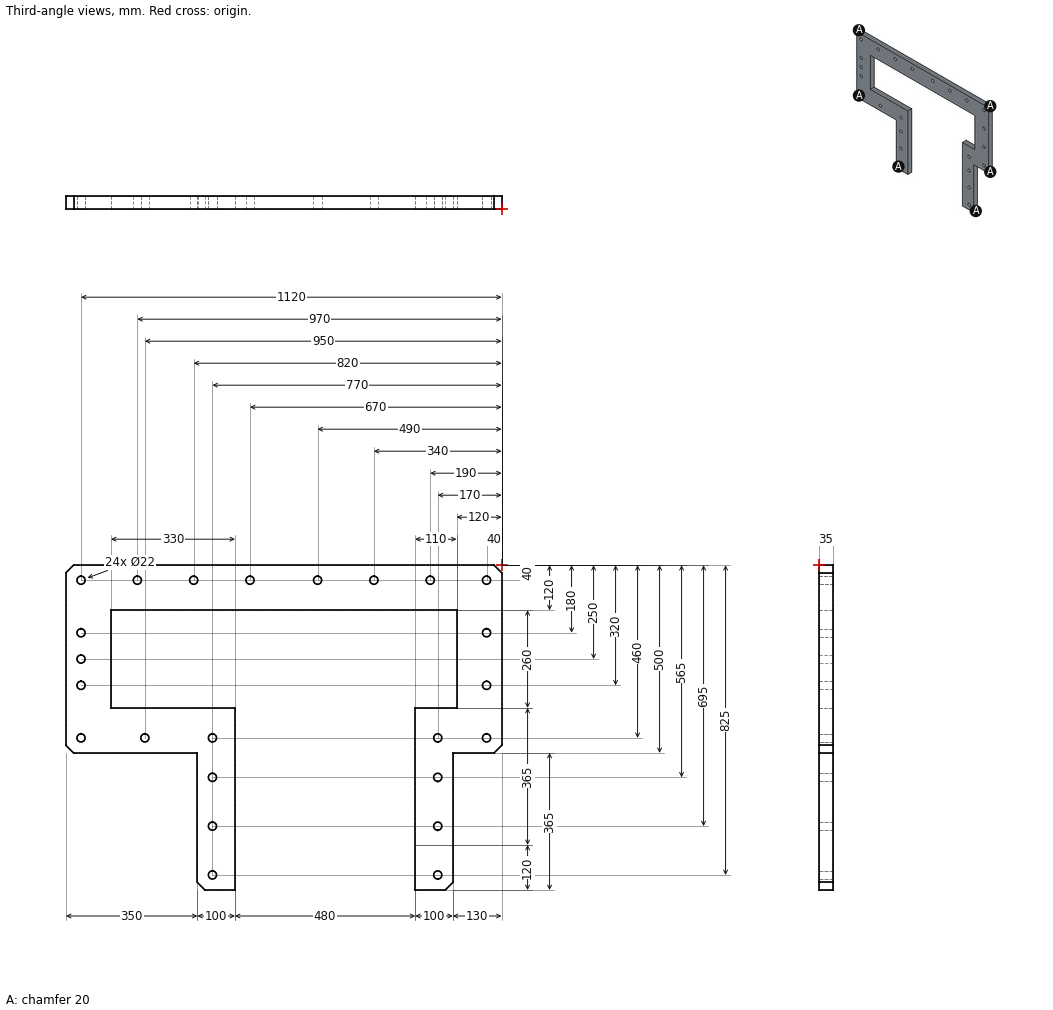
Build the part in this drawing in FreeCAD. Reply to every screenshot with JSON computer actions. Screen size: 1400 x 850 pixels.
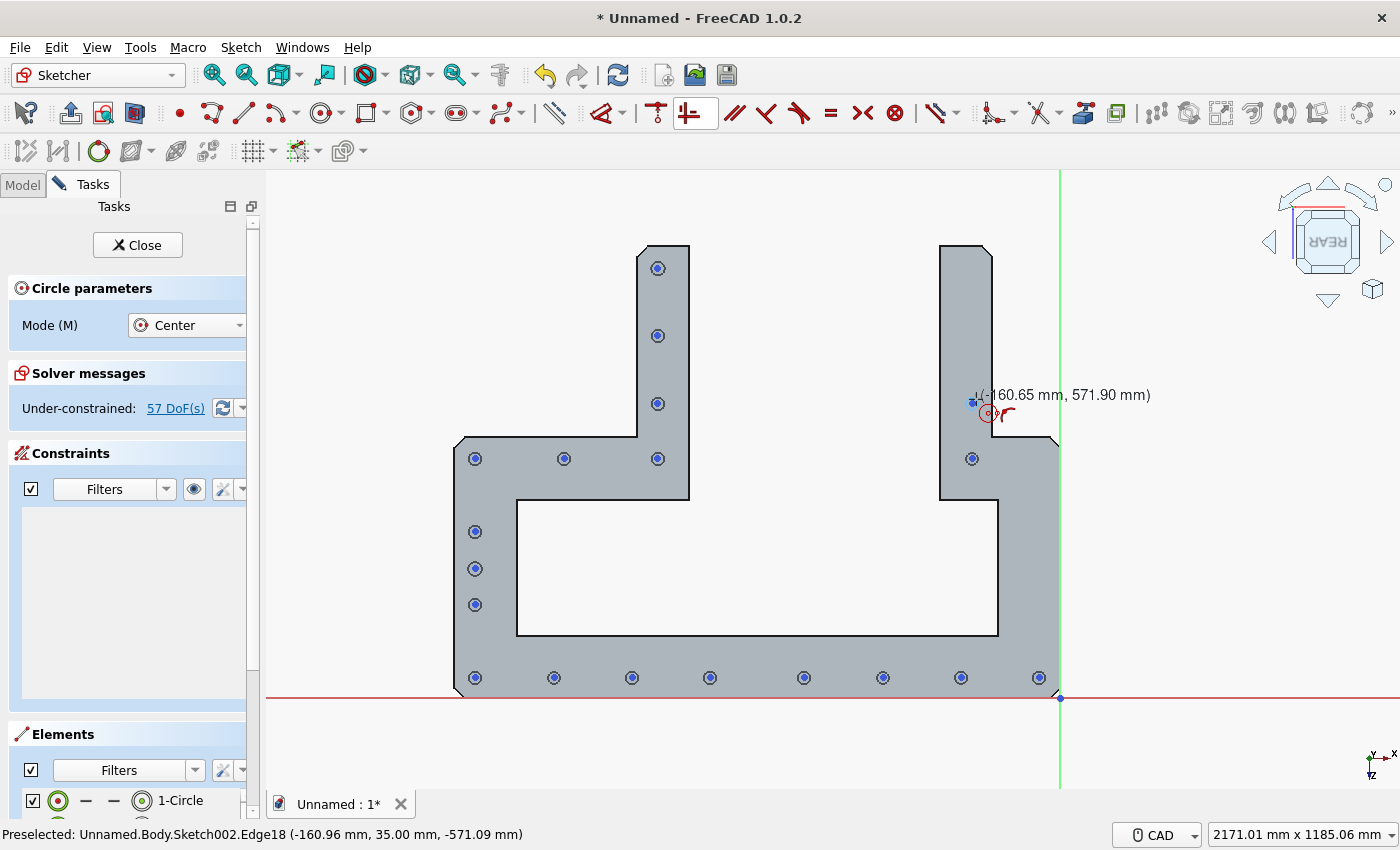
{"action": "scroll", "coordinate": [972, 335], "scroll_direction": "up", "scroll_amount": 7}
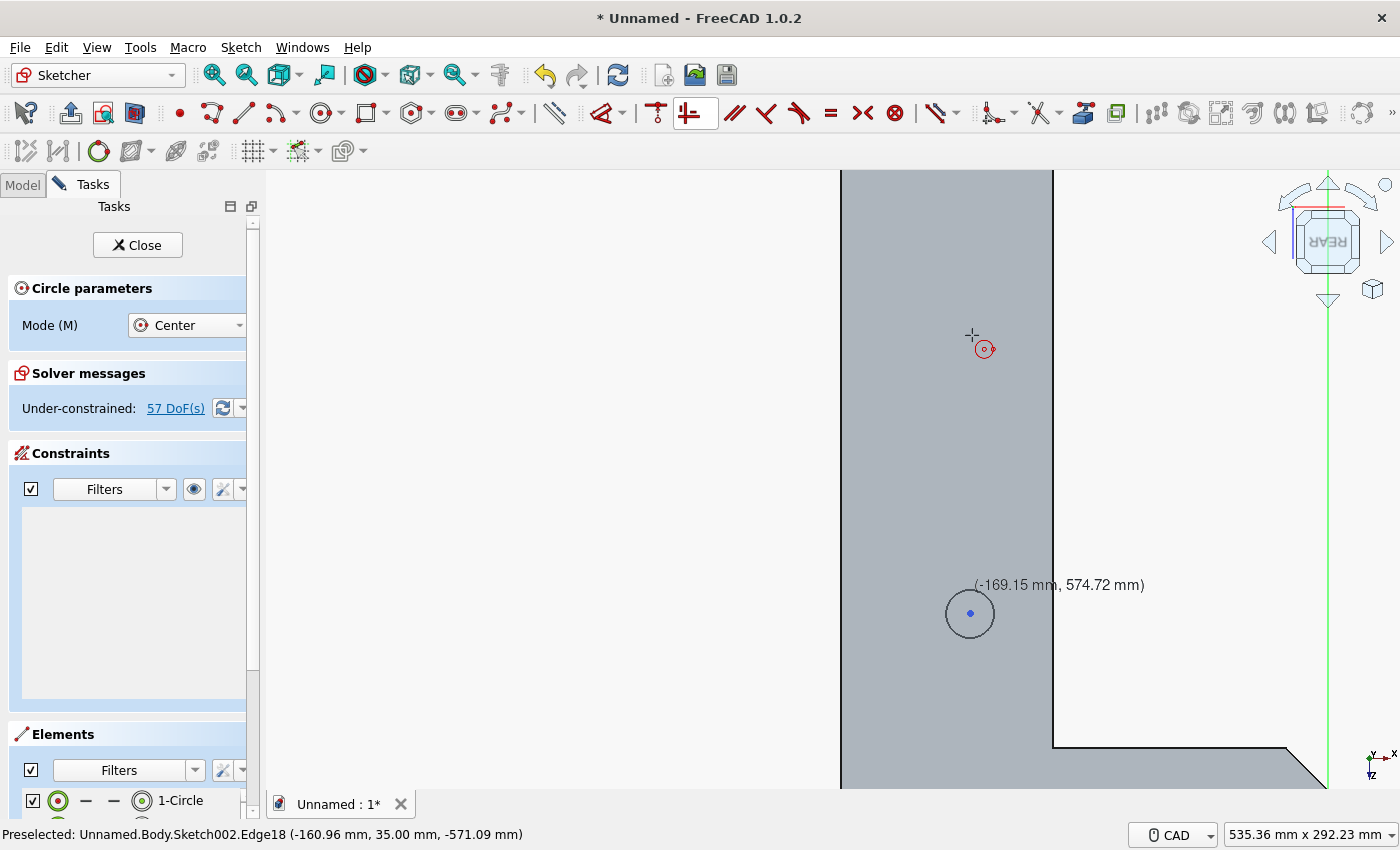
{"action": "scroll", "coordinate": [972, 335], "scroll_direction": "down", "scroll_amount": 7}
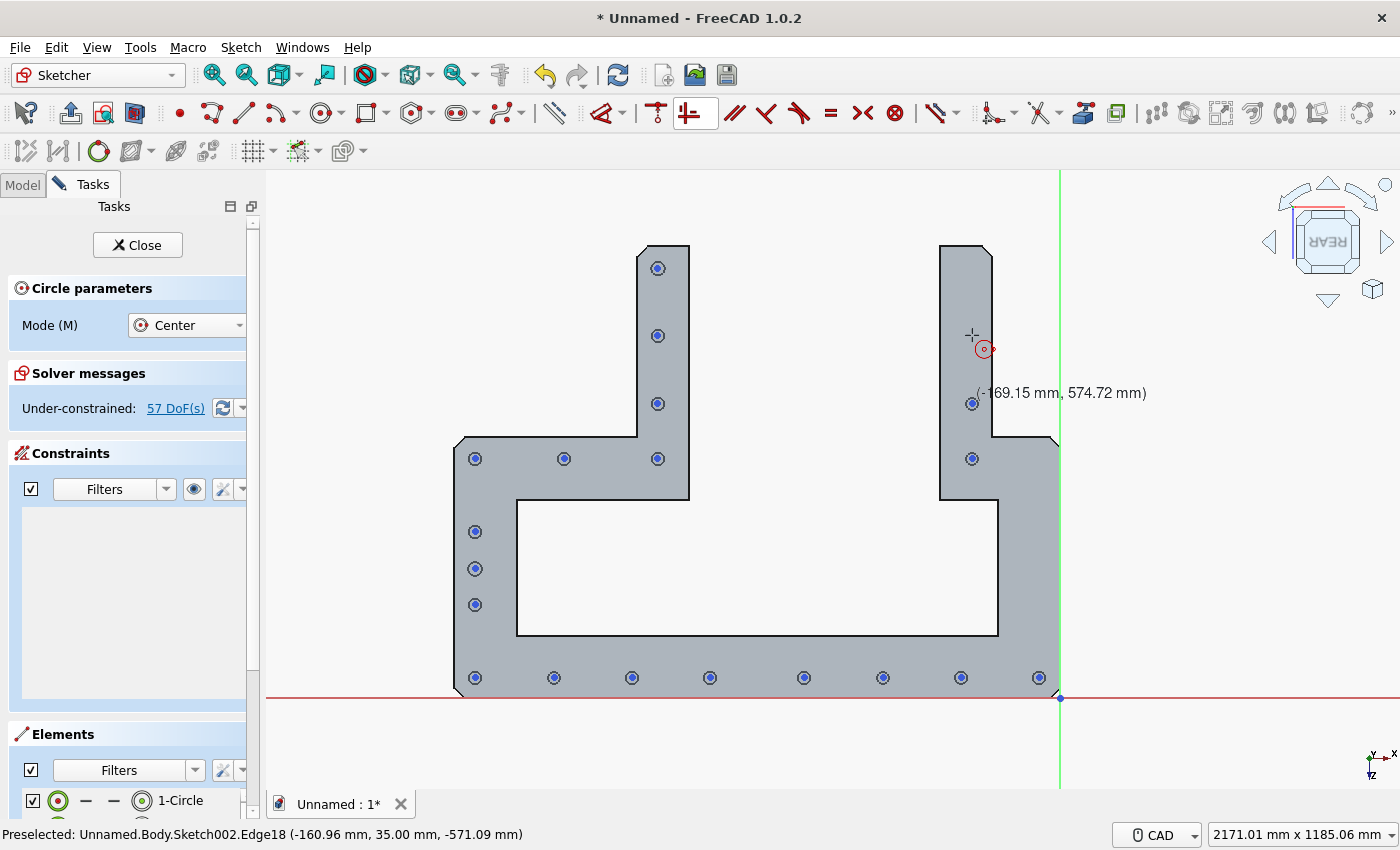
{"action": "left_click", "coordinate": [972, 335]}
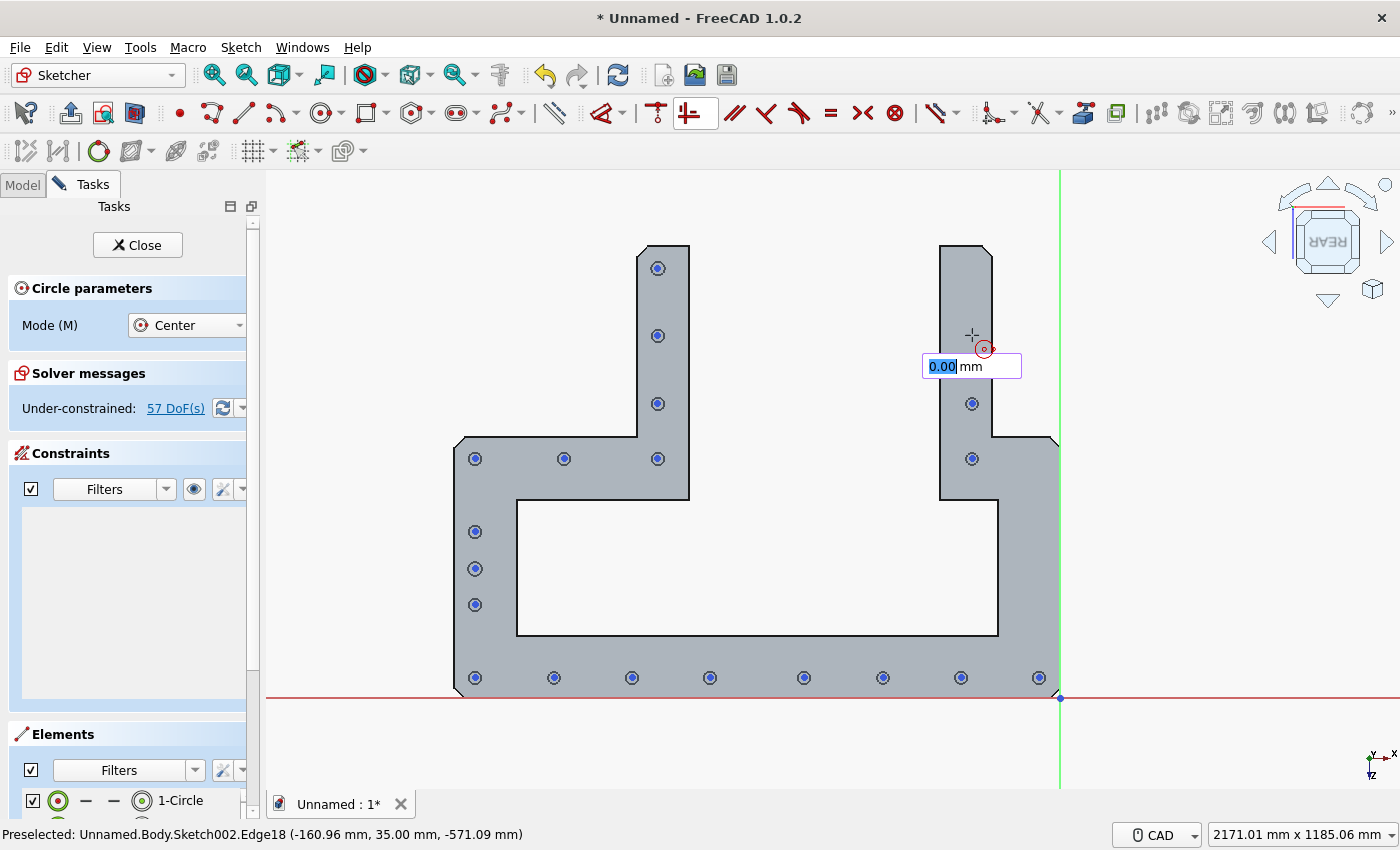
{"action": "scroll", "coordinate": [976, 331], "scroll_direction": "up", "scroll_amount": 6}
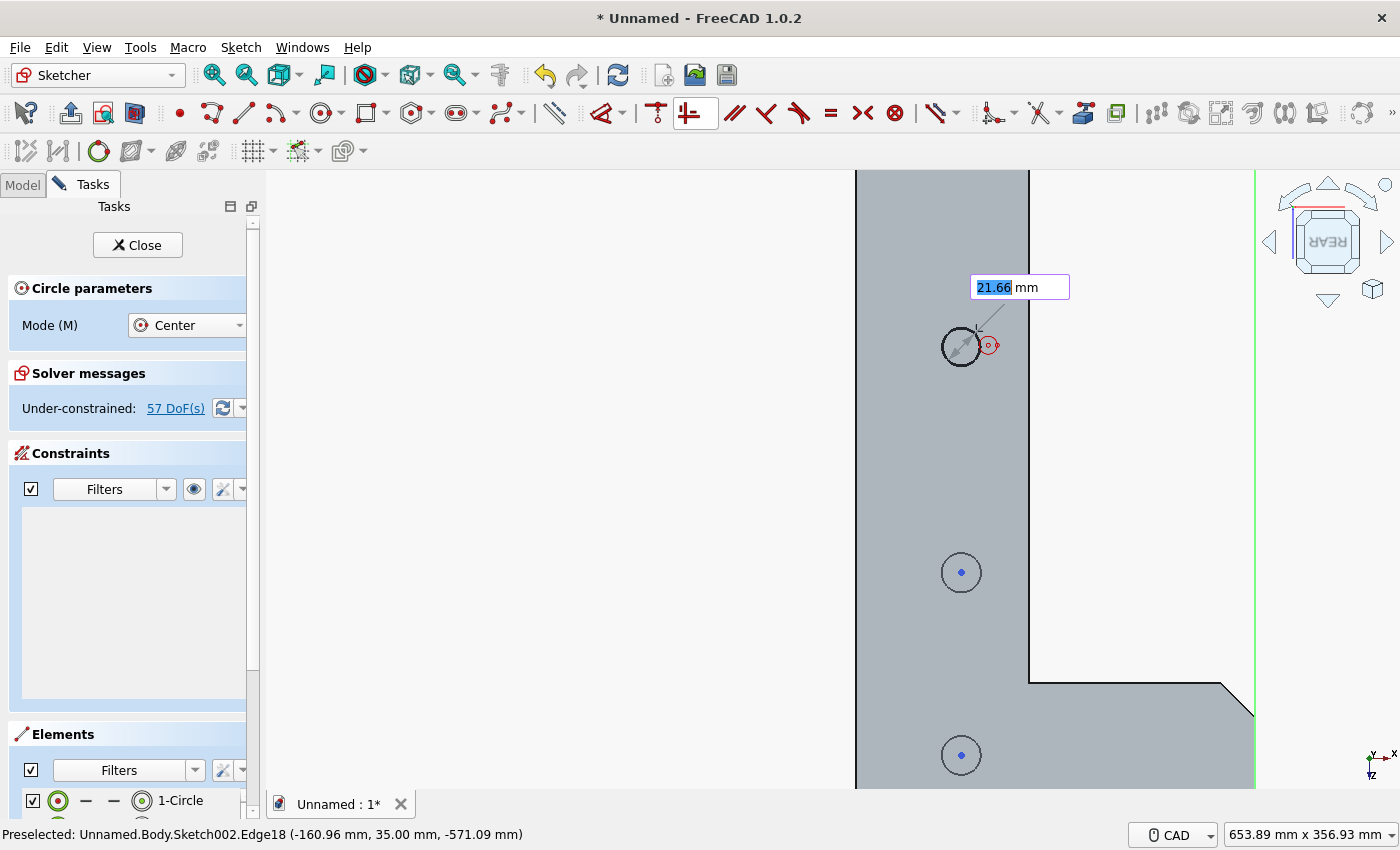
{"action": "left_click", "coordinate": [973, 331]}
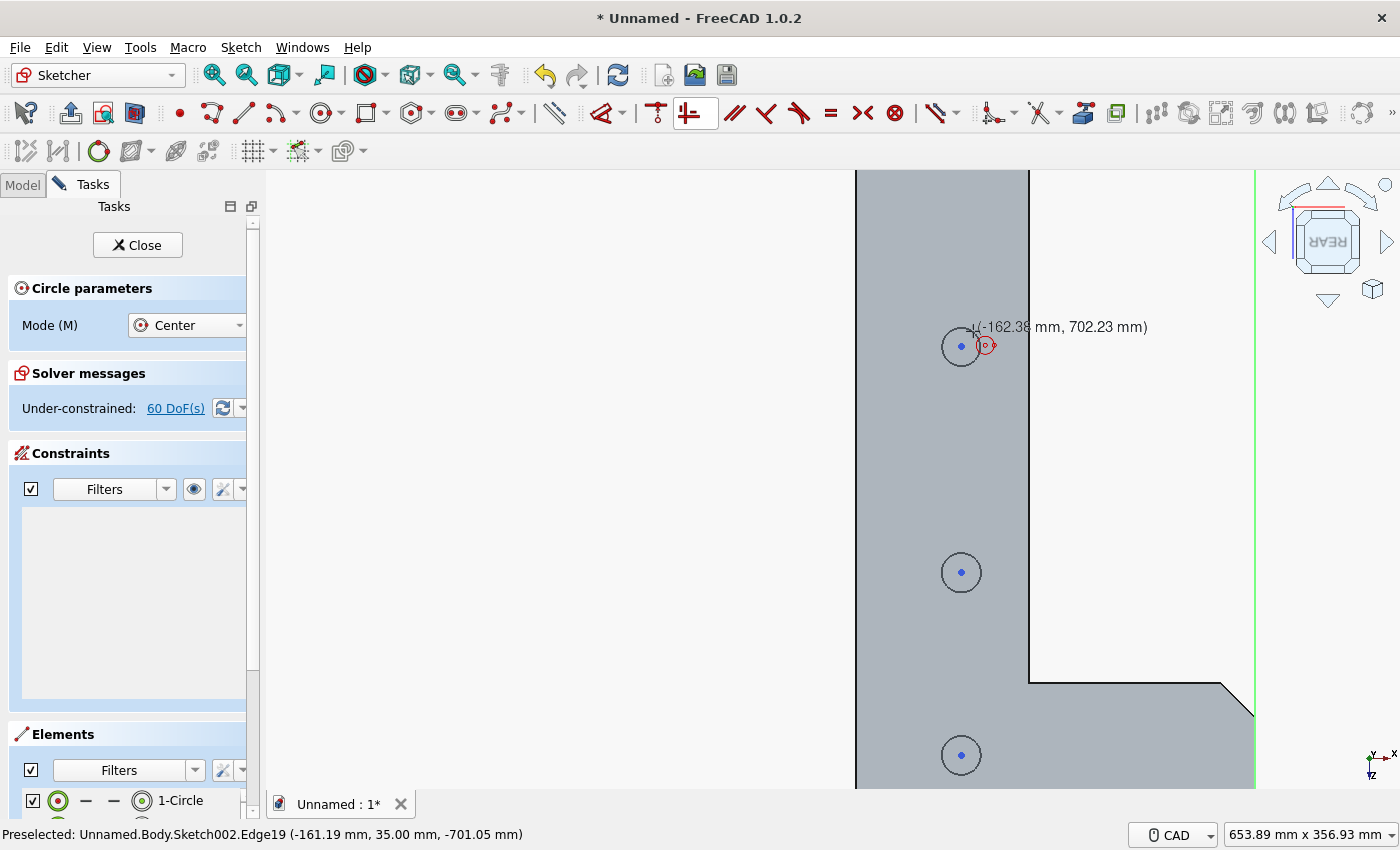
{"action": "scroll", "coordinate": [976, 331], "scroll_direction": "down", "scroll_amount": 6}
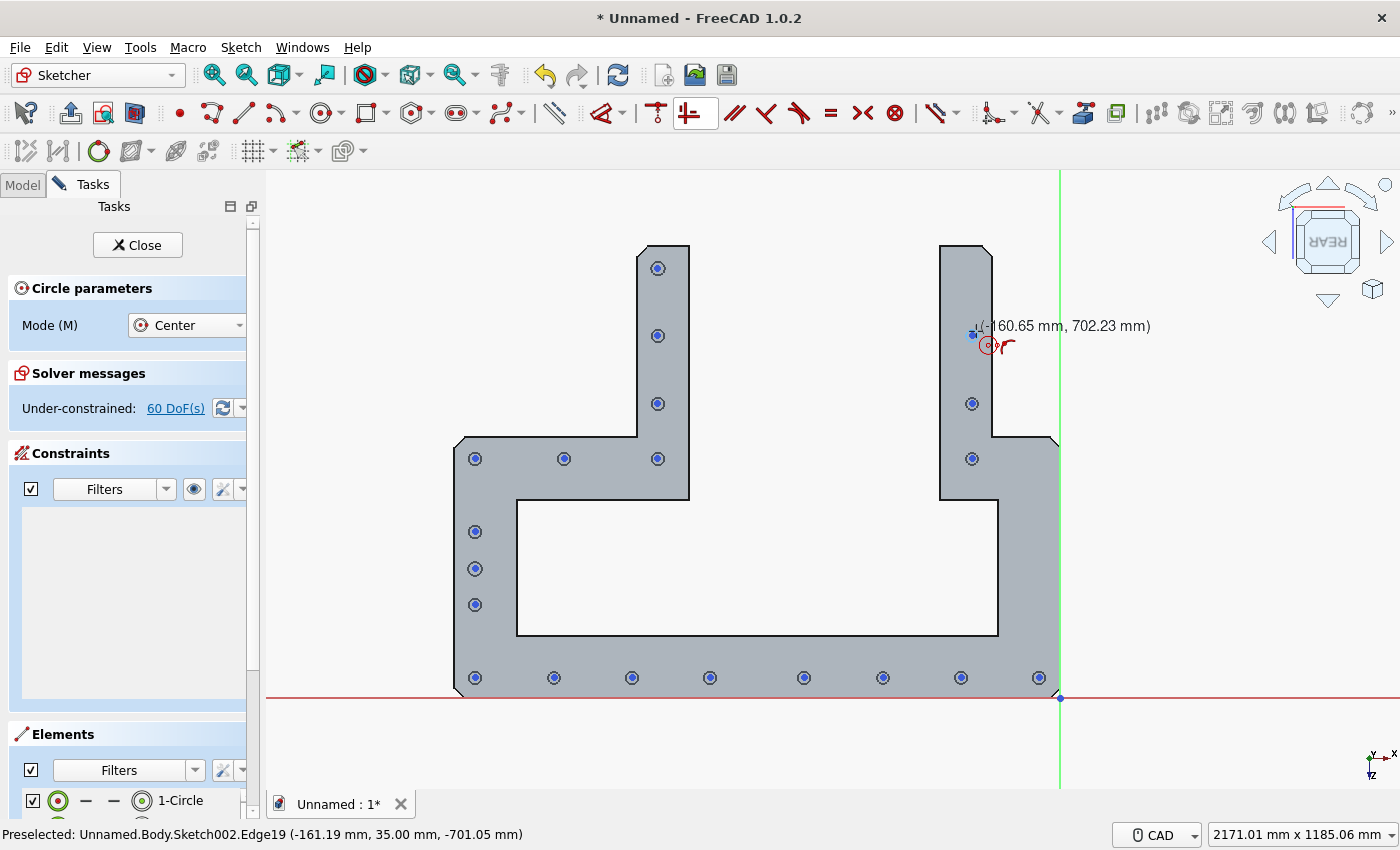
{"action": "scroll", "coordinate": [972, 267], "scroll_direction": "up", "scroll_amount": 7}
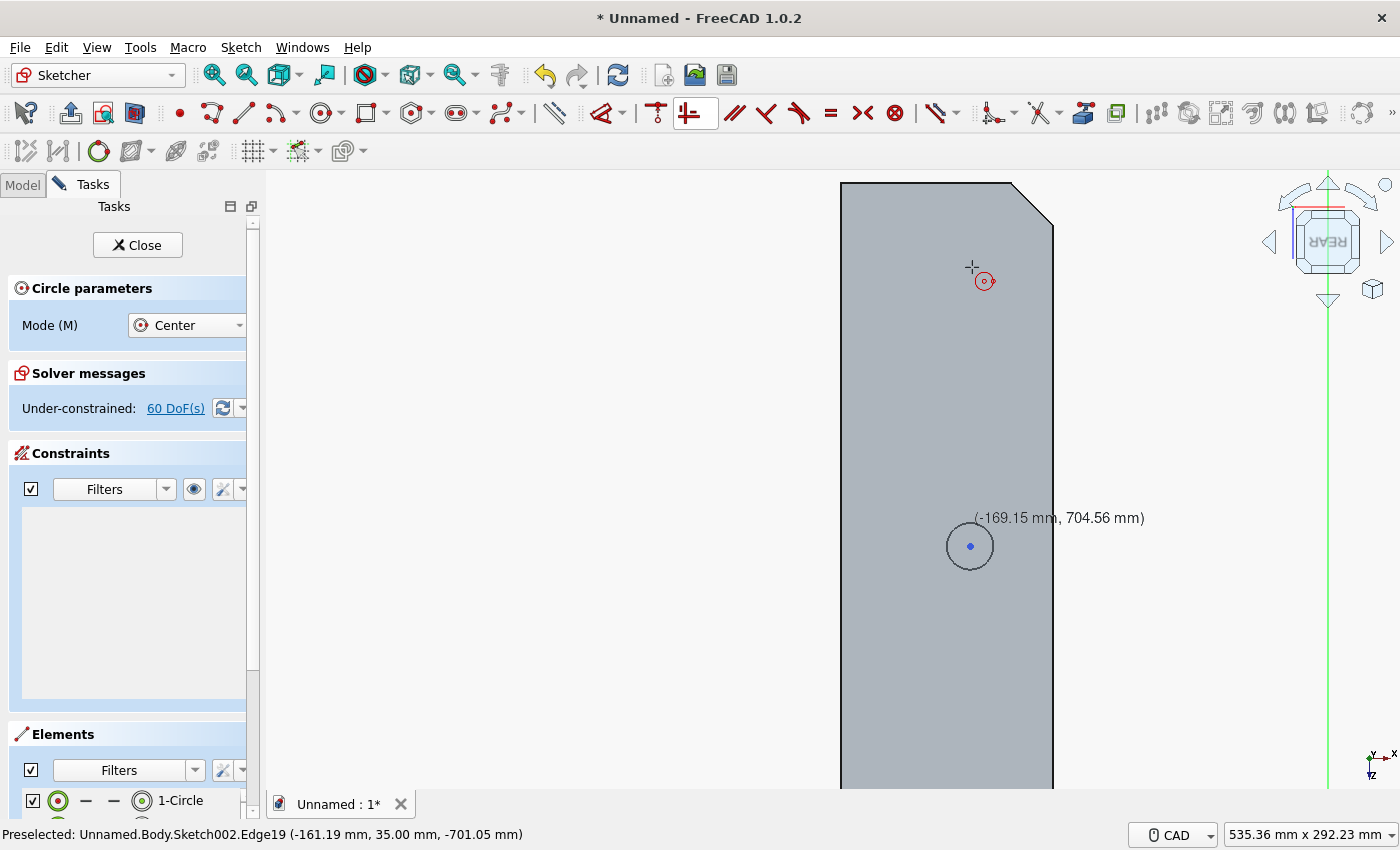
{"action": "scroll", "coordinate": [972, 267], "scroll_direction": "down", "scroll_amount": 7}